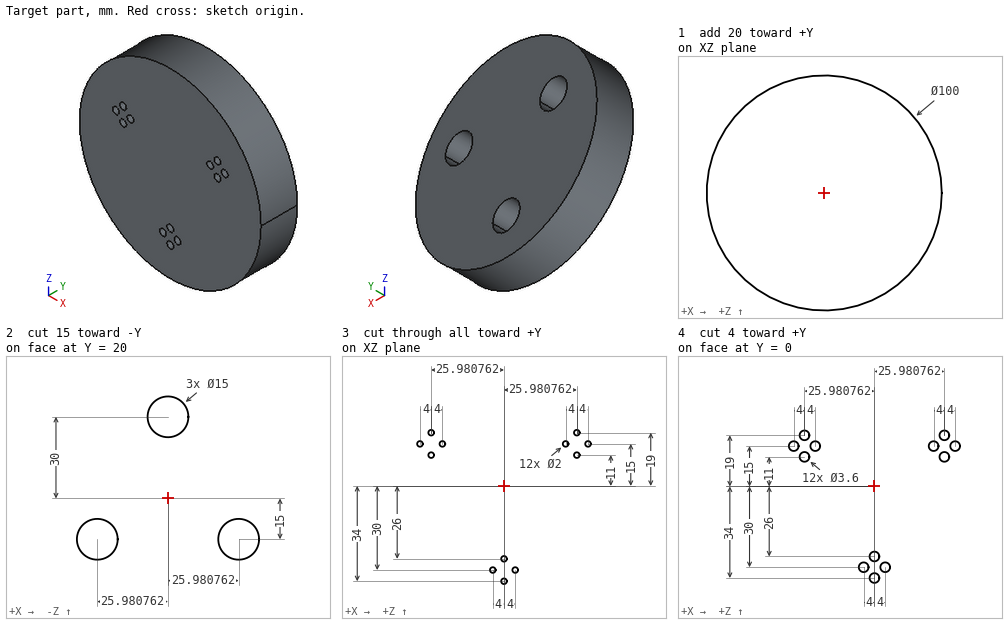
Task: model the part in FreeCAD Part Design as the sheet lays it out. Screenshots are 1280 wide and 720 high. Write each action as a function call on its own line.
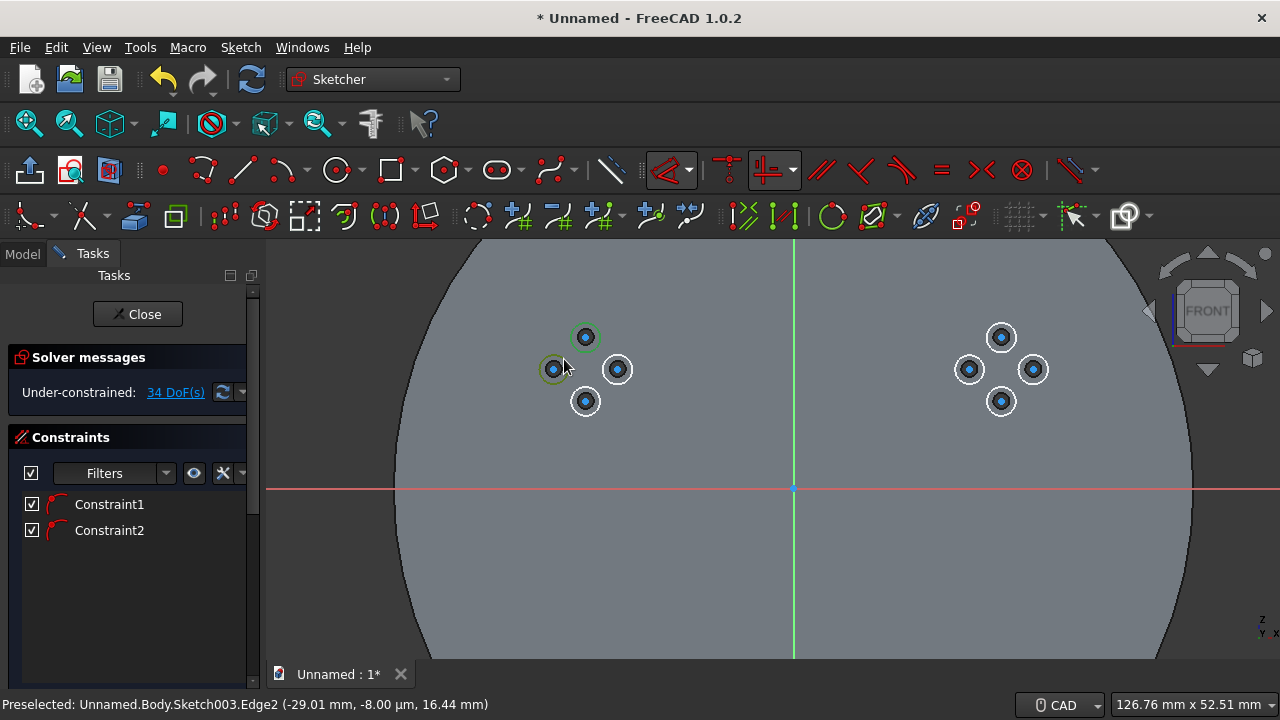
click(596, 391)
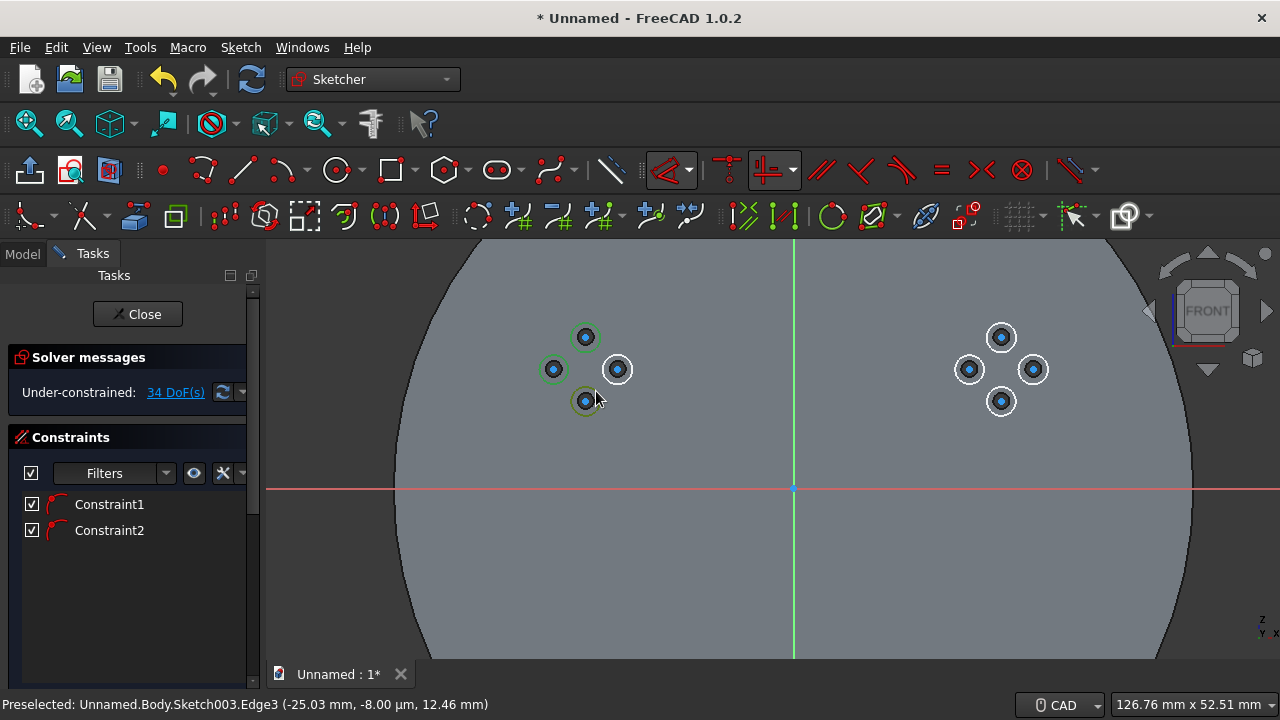
click(628, 359)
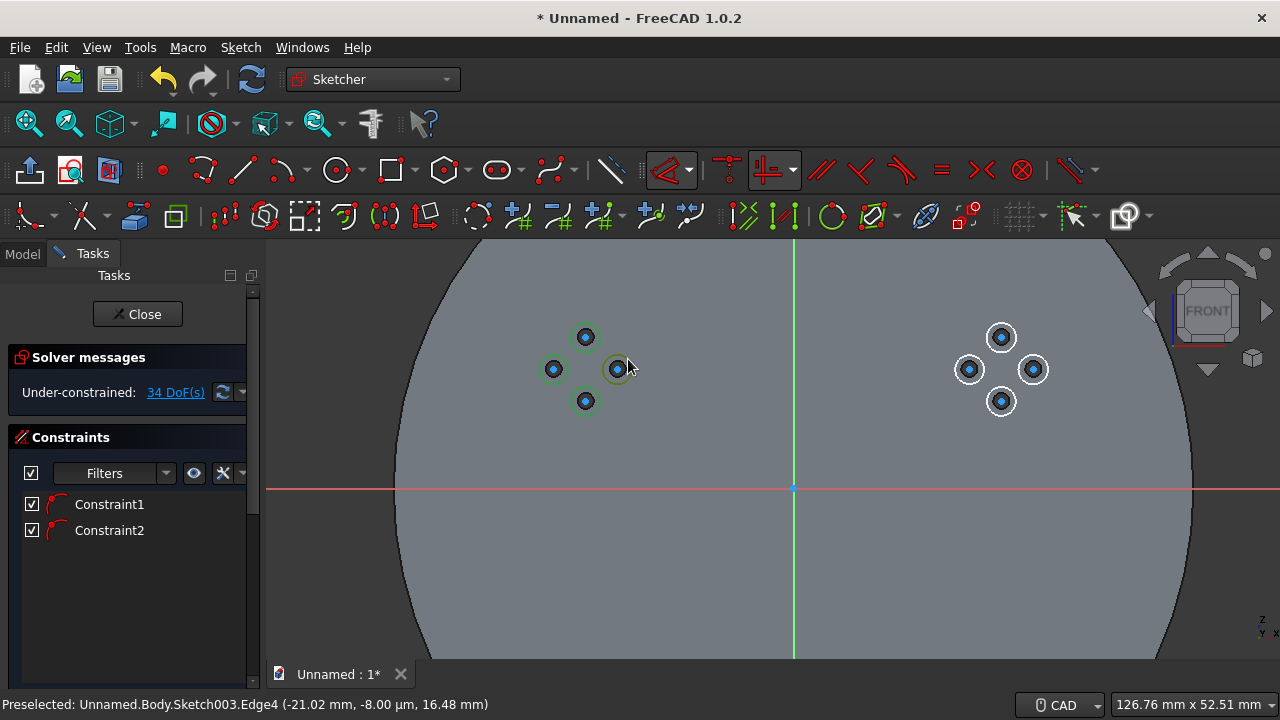
click(1012, 327)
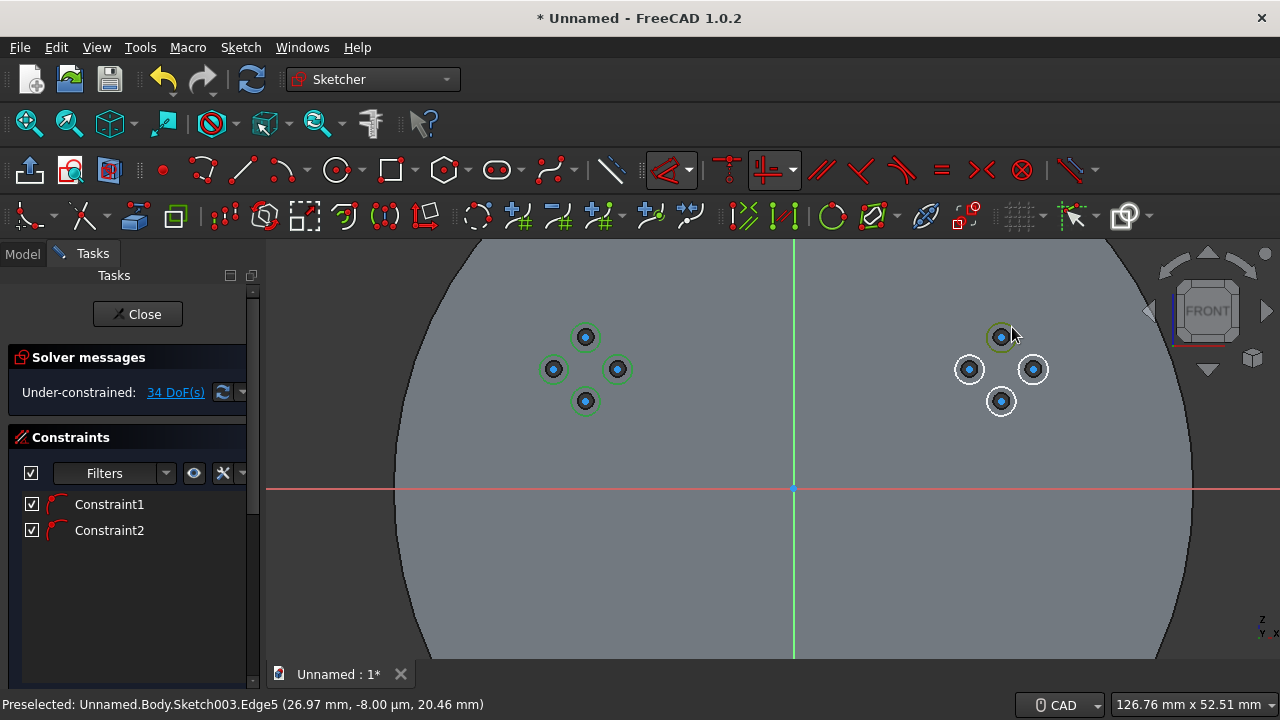
click(980, 359)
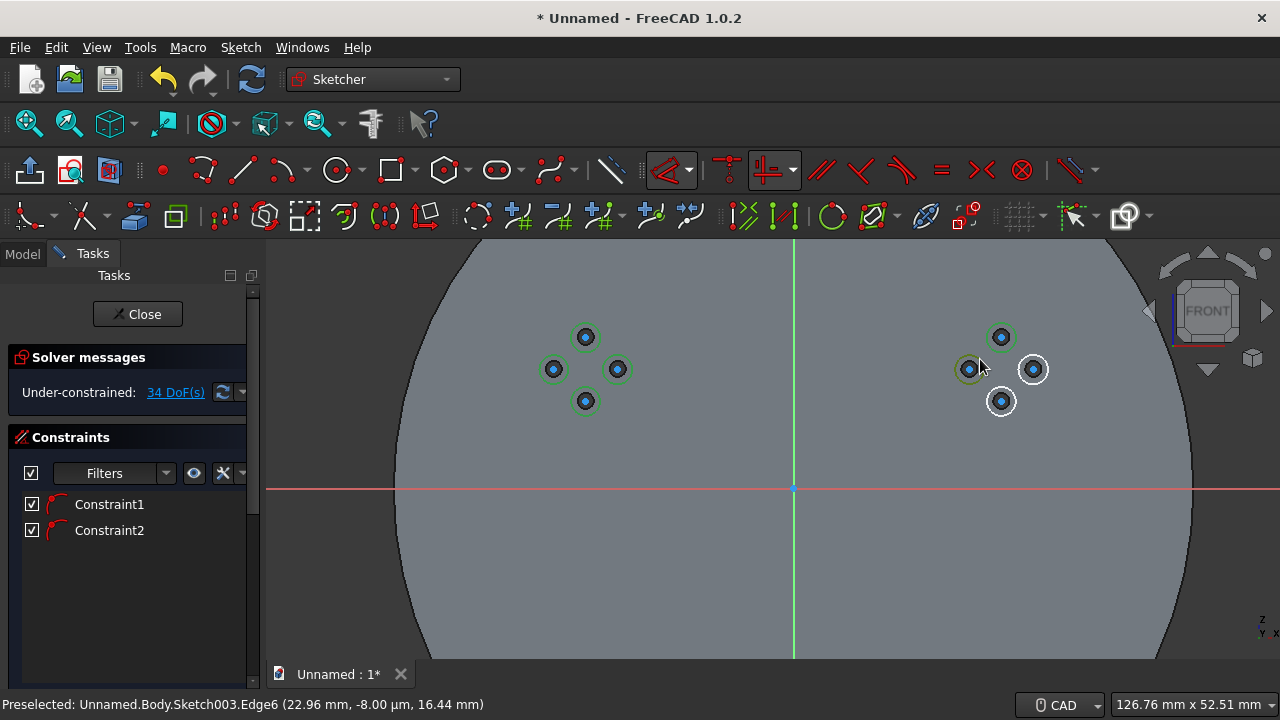
click(1012, 391)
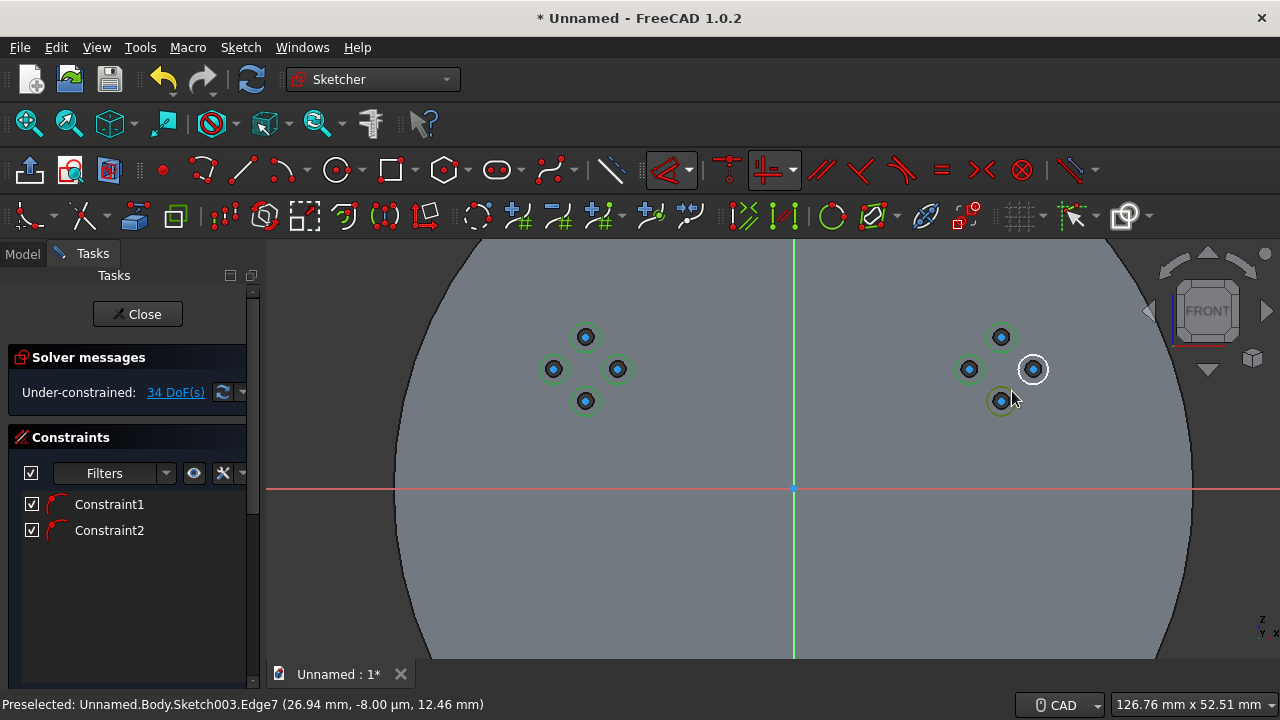
click(1044, 359)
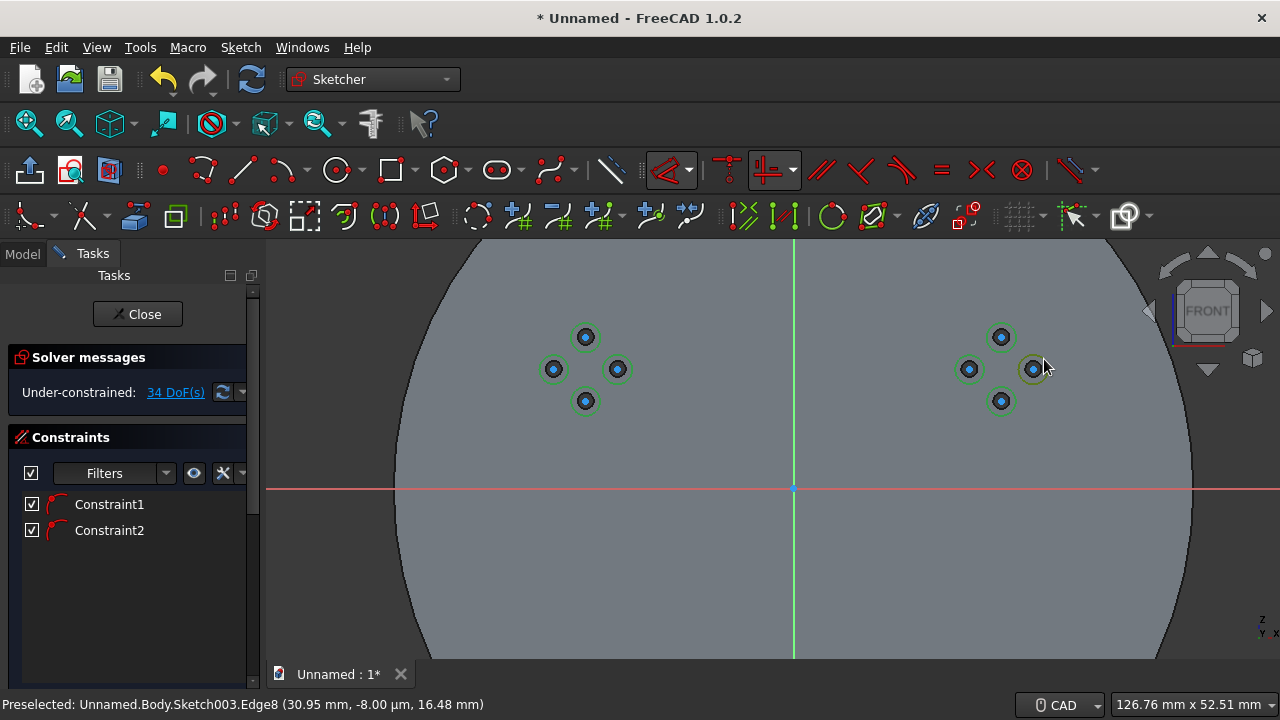
scroll(596, 327, down, 3)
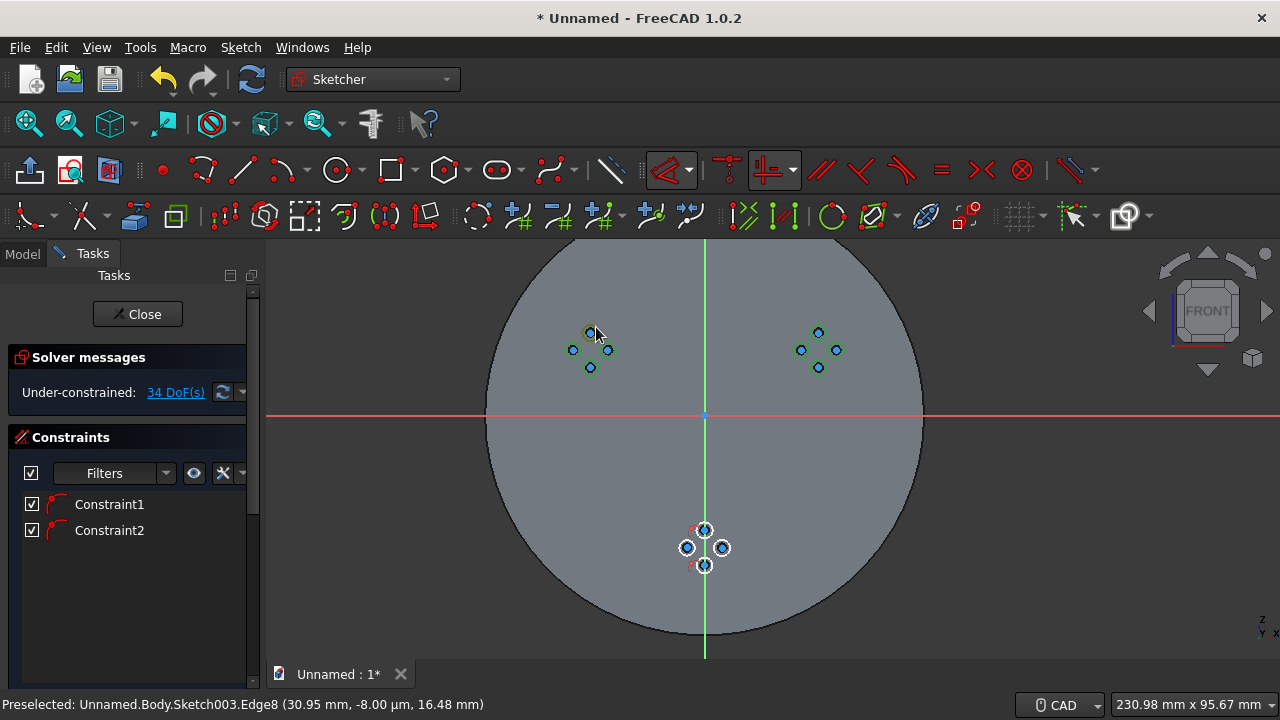
scroll(710, 525, up, 5)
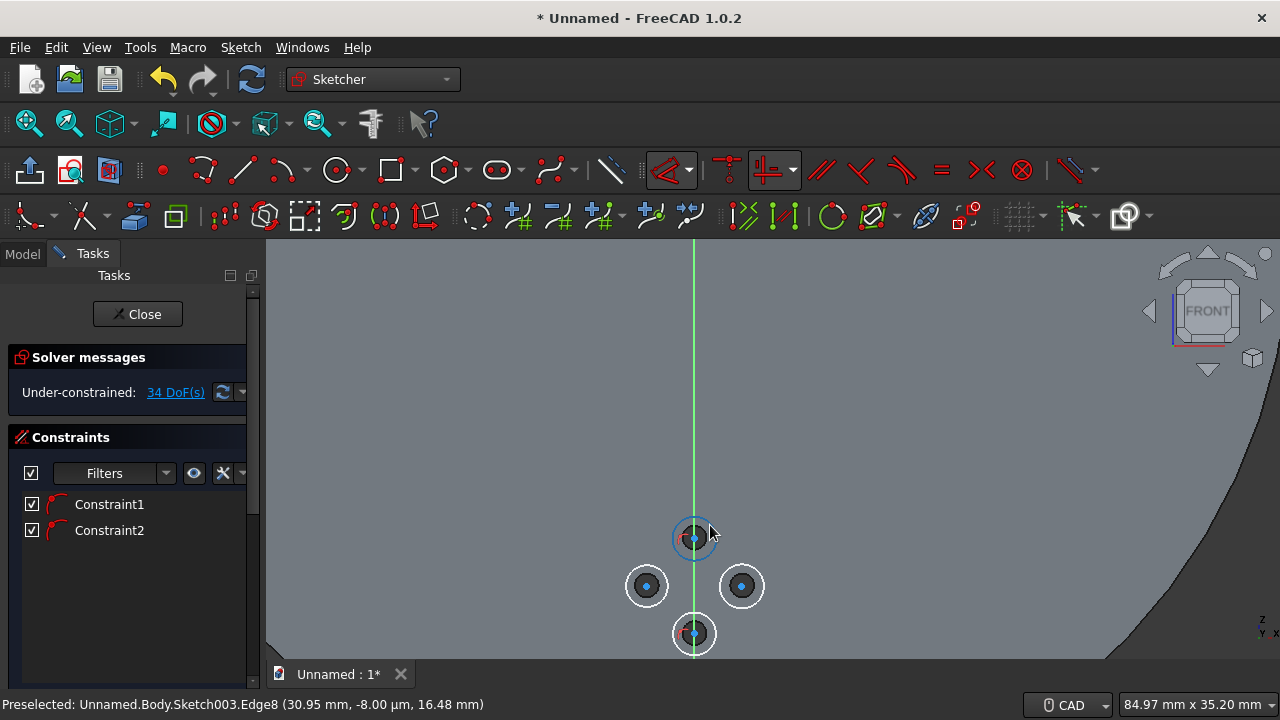
click(710, 523)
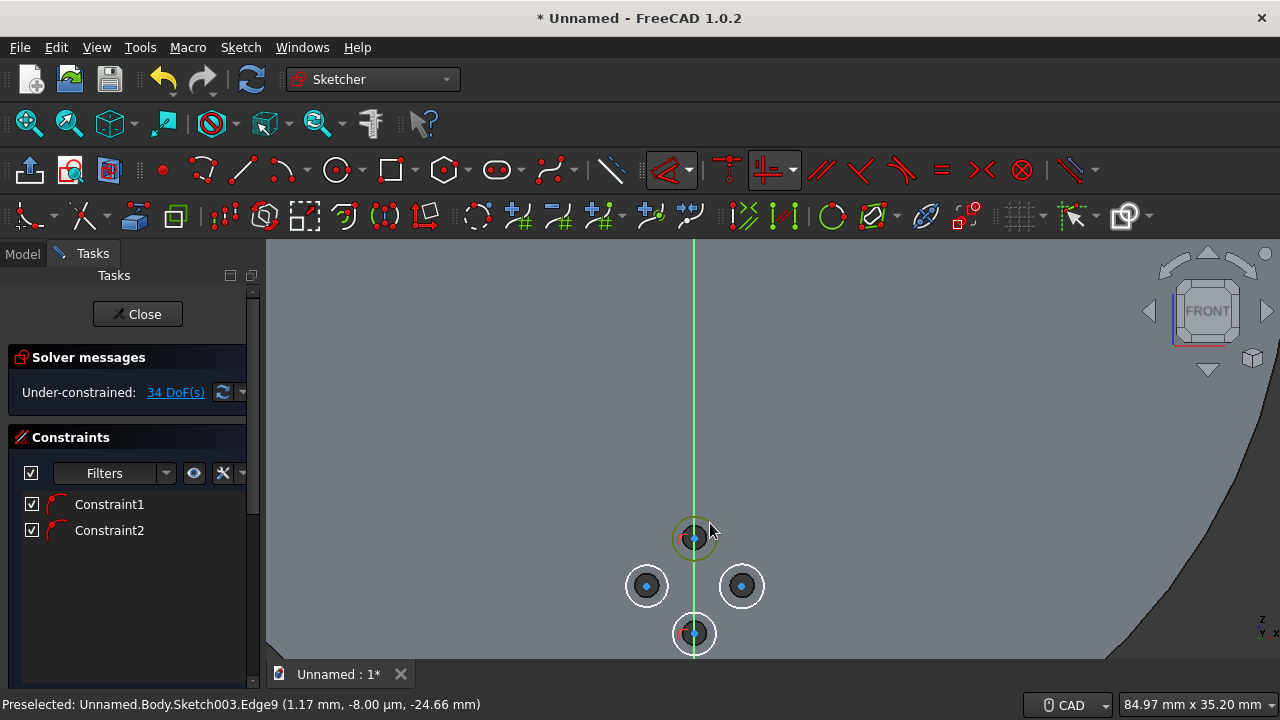
click(662, 571)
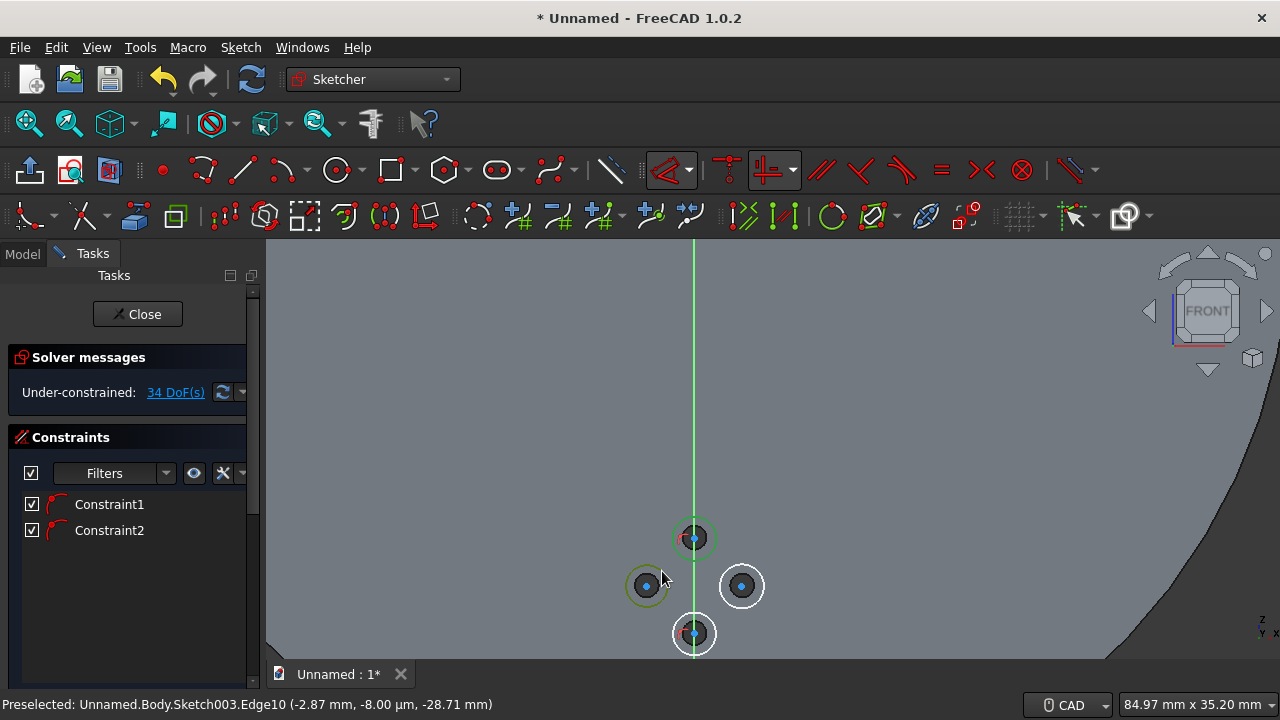
click(710, 619)